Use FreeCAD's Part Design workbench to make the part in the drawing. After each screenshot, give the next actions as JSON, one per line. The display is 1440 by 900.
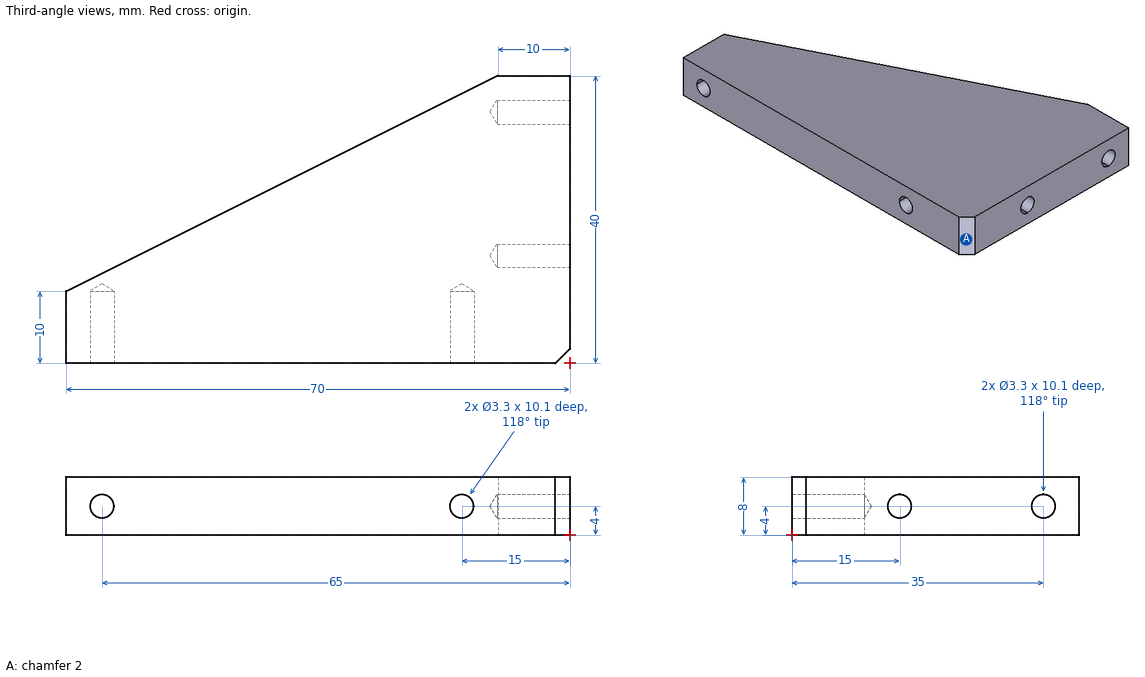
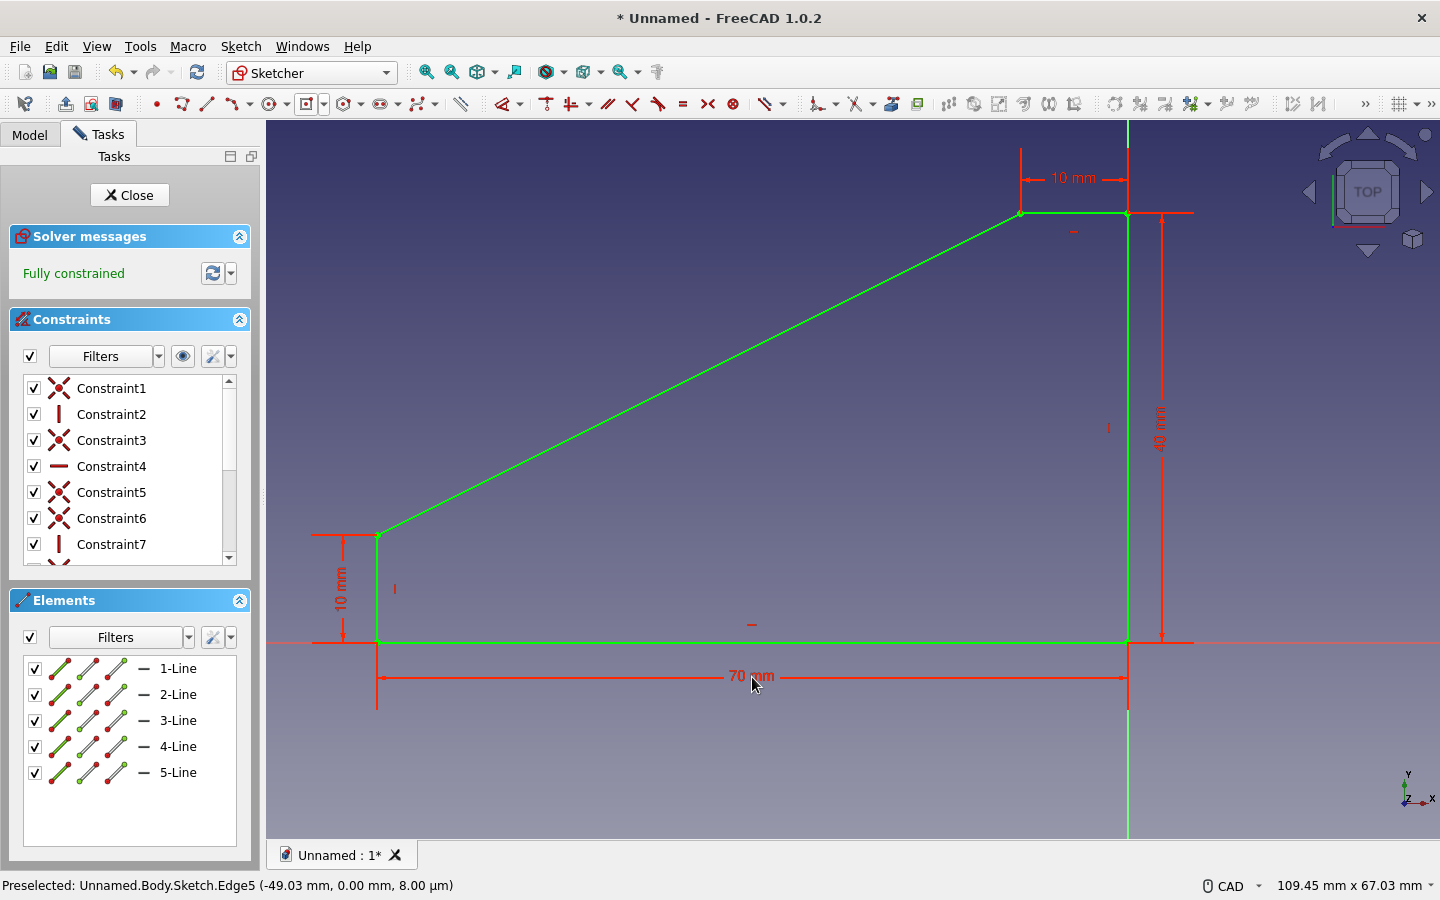
{"action": "left_click", "coordinate": [130, 195]}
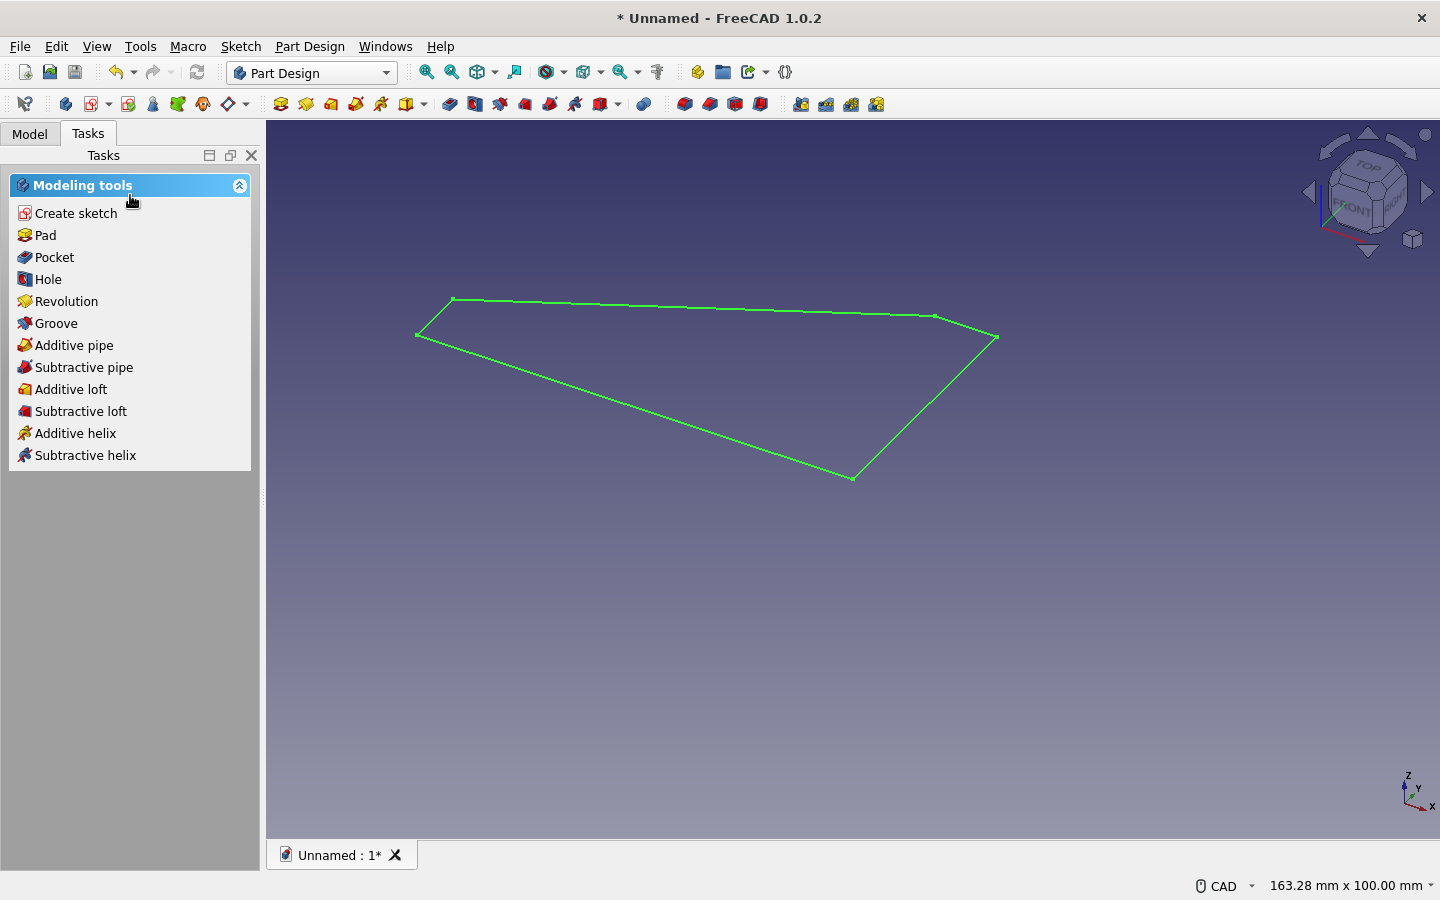
{"action": "left_click", "coordinate": [281, 104]}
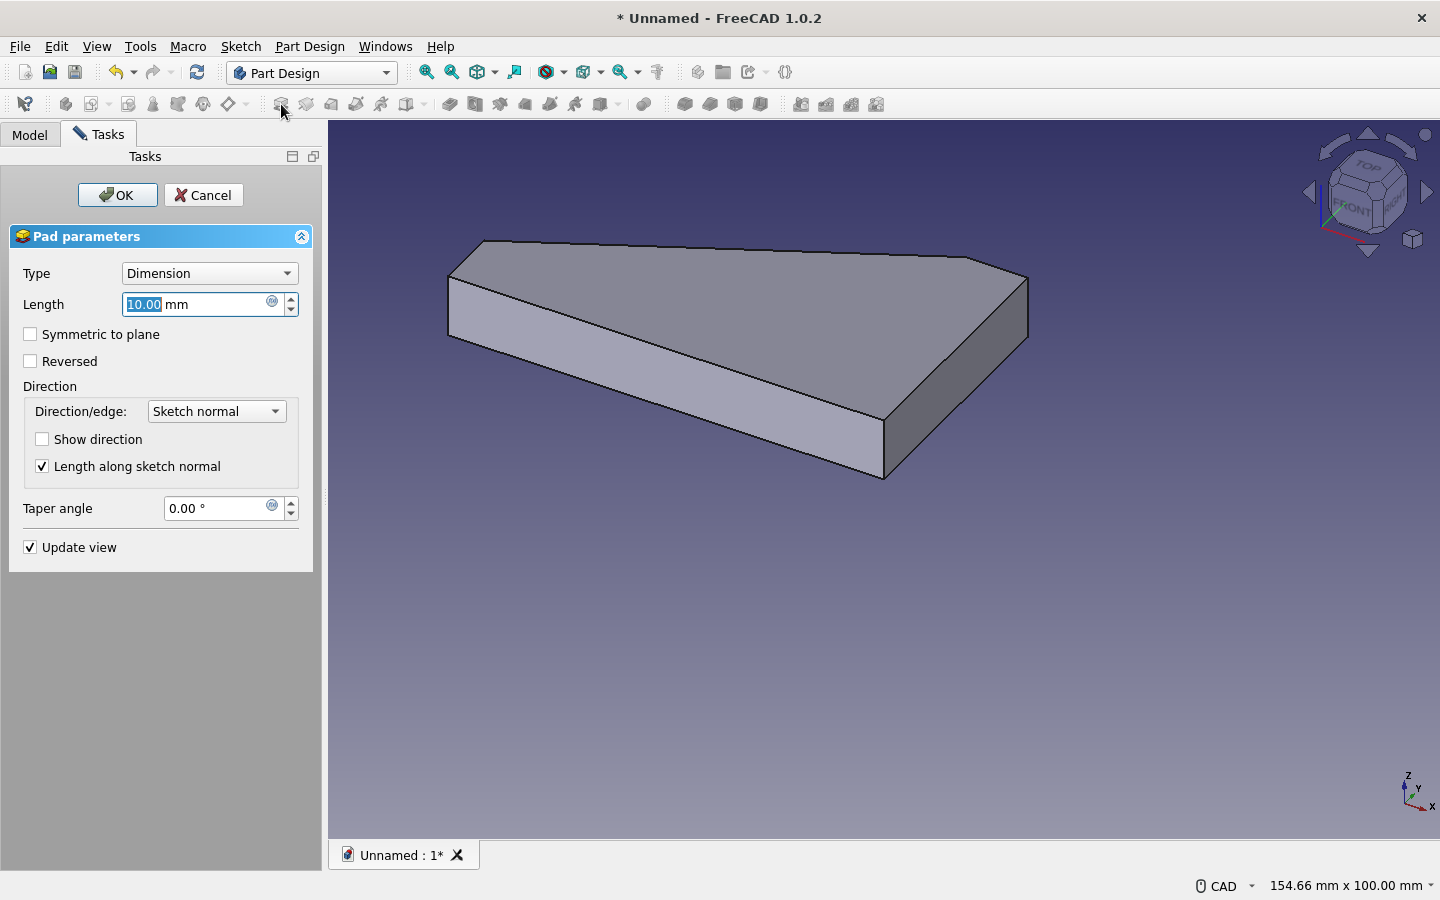
{"action": "type", "text": "8"}
{"action": "key", "text": "Tab"}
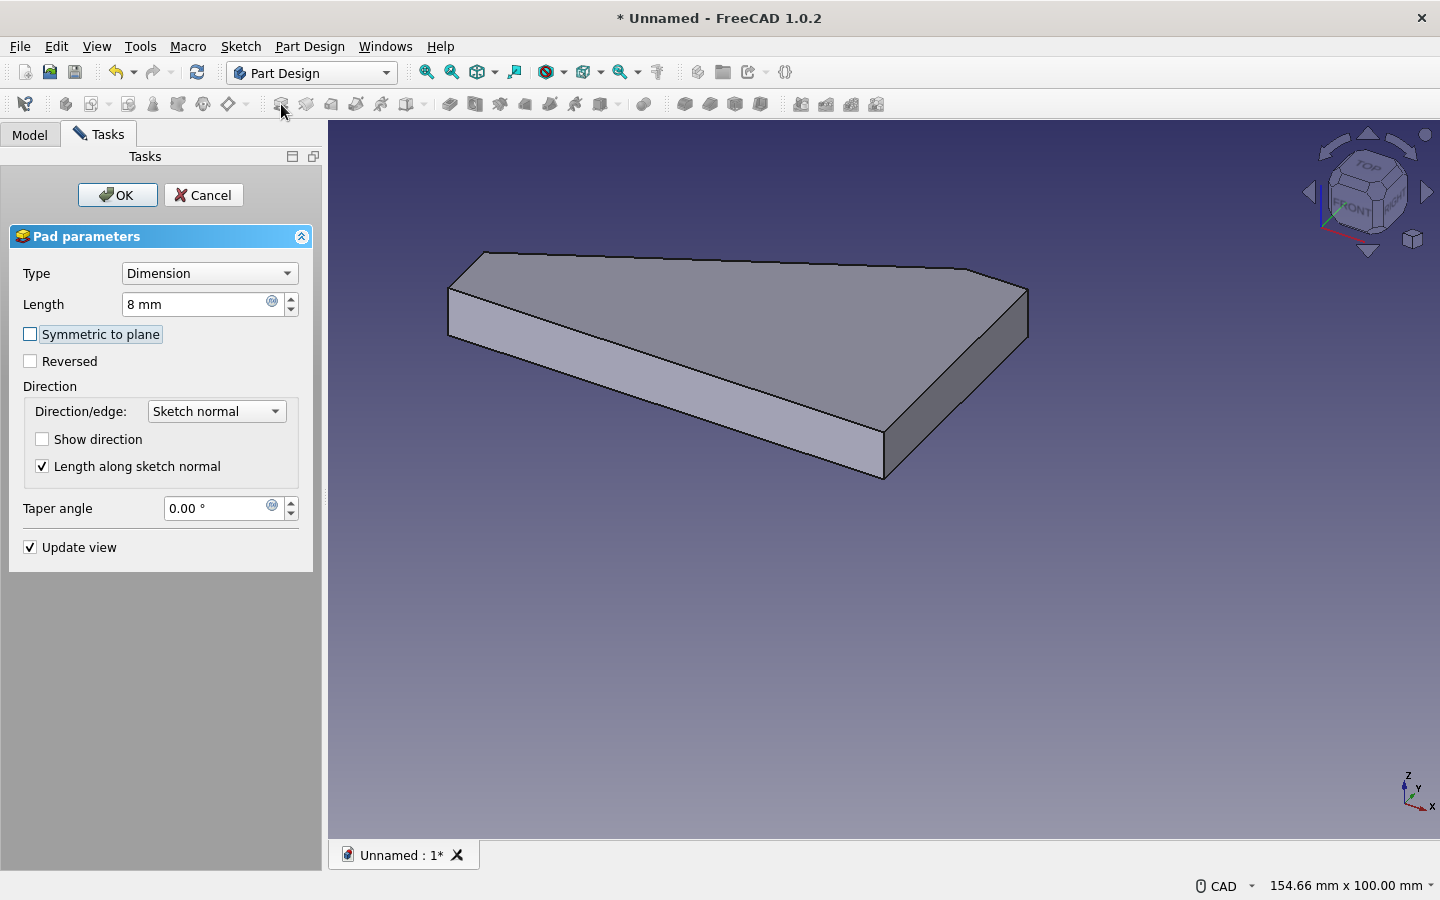
{"action": "left_click", "coordinate": [118, 195]}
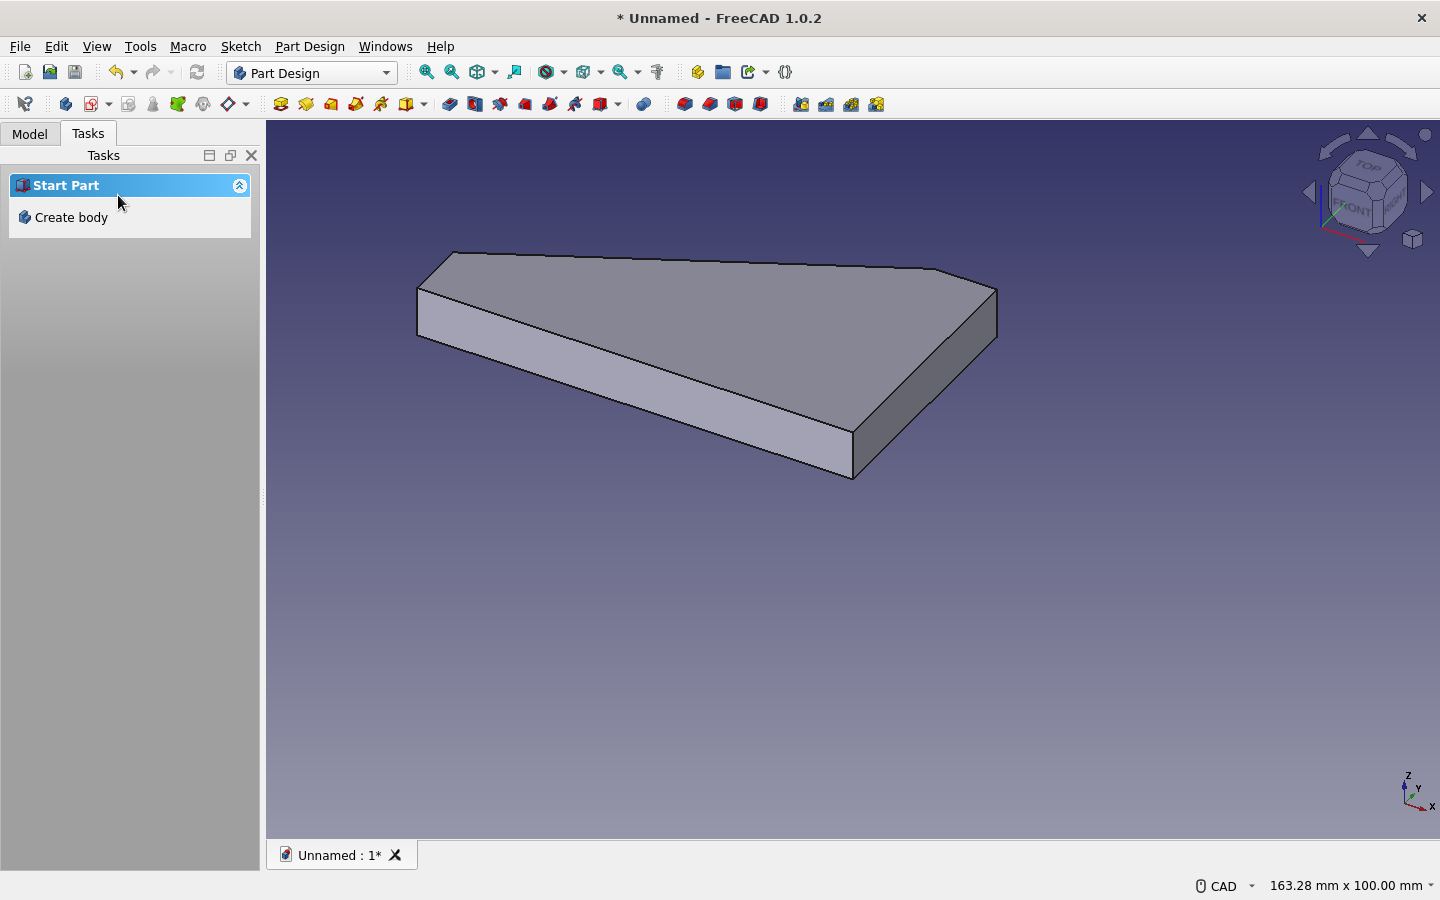
{"action": "left_click", "coordinate": [90, 104]}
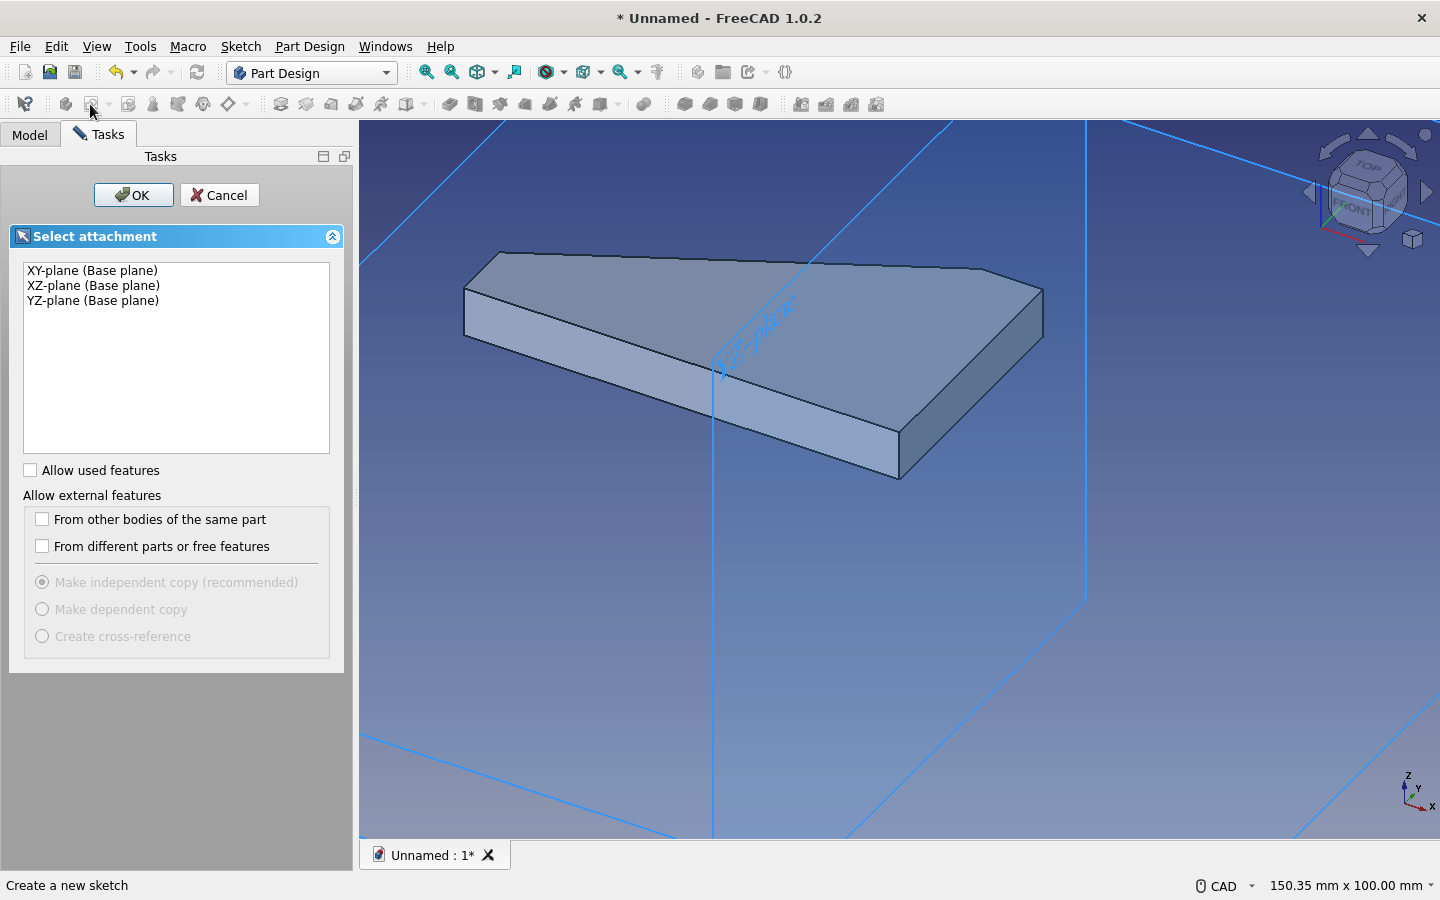
{"action": "left_click", "coordinate": [84, 286]}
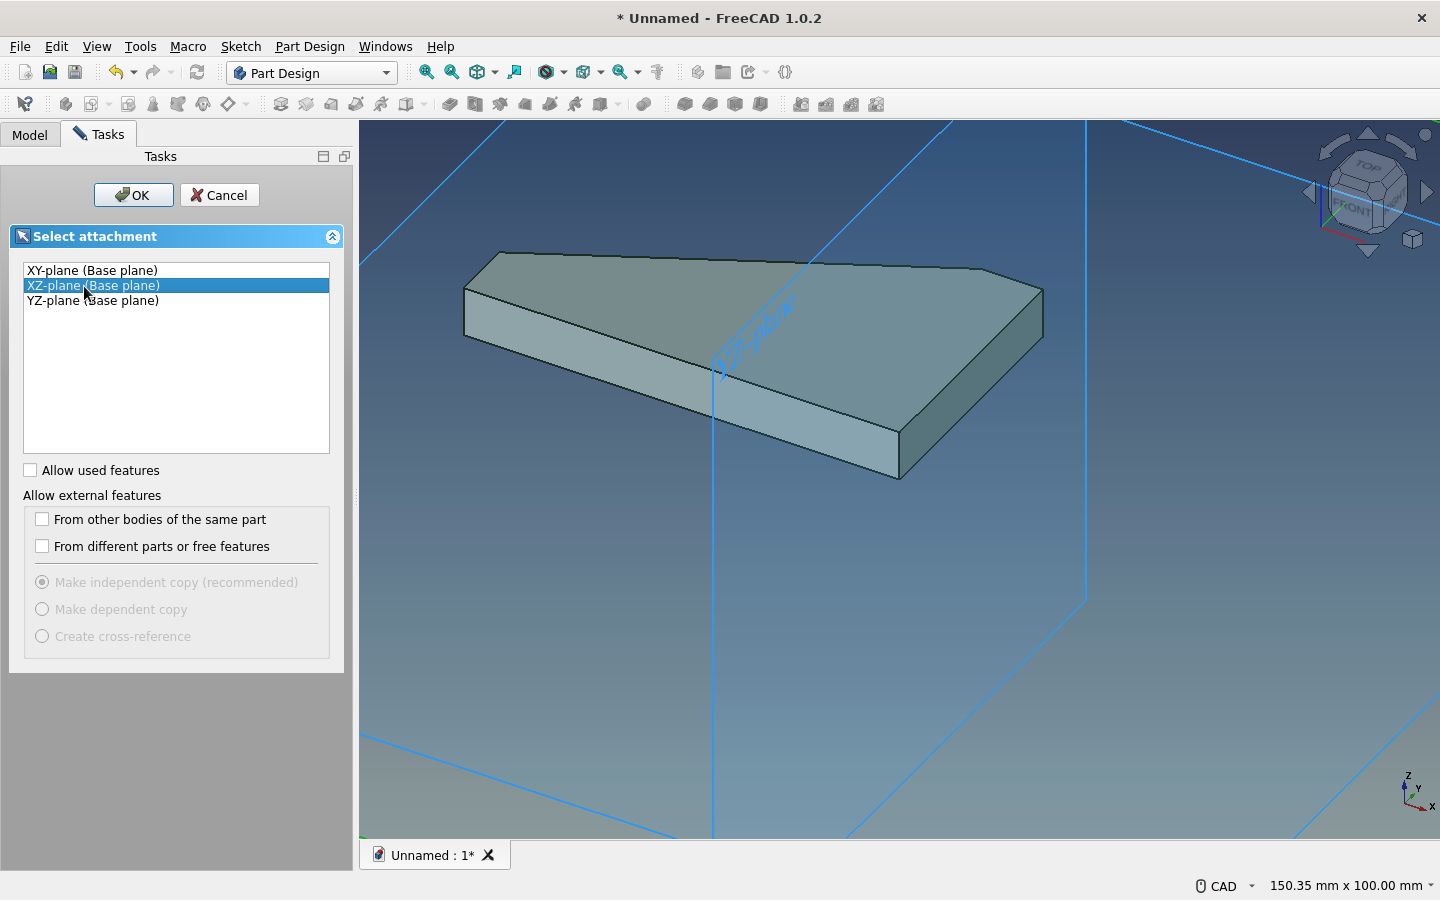
{"action": "left_click", "coordinate": [134, 195]}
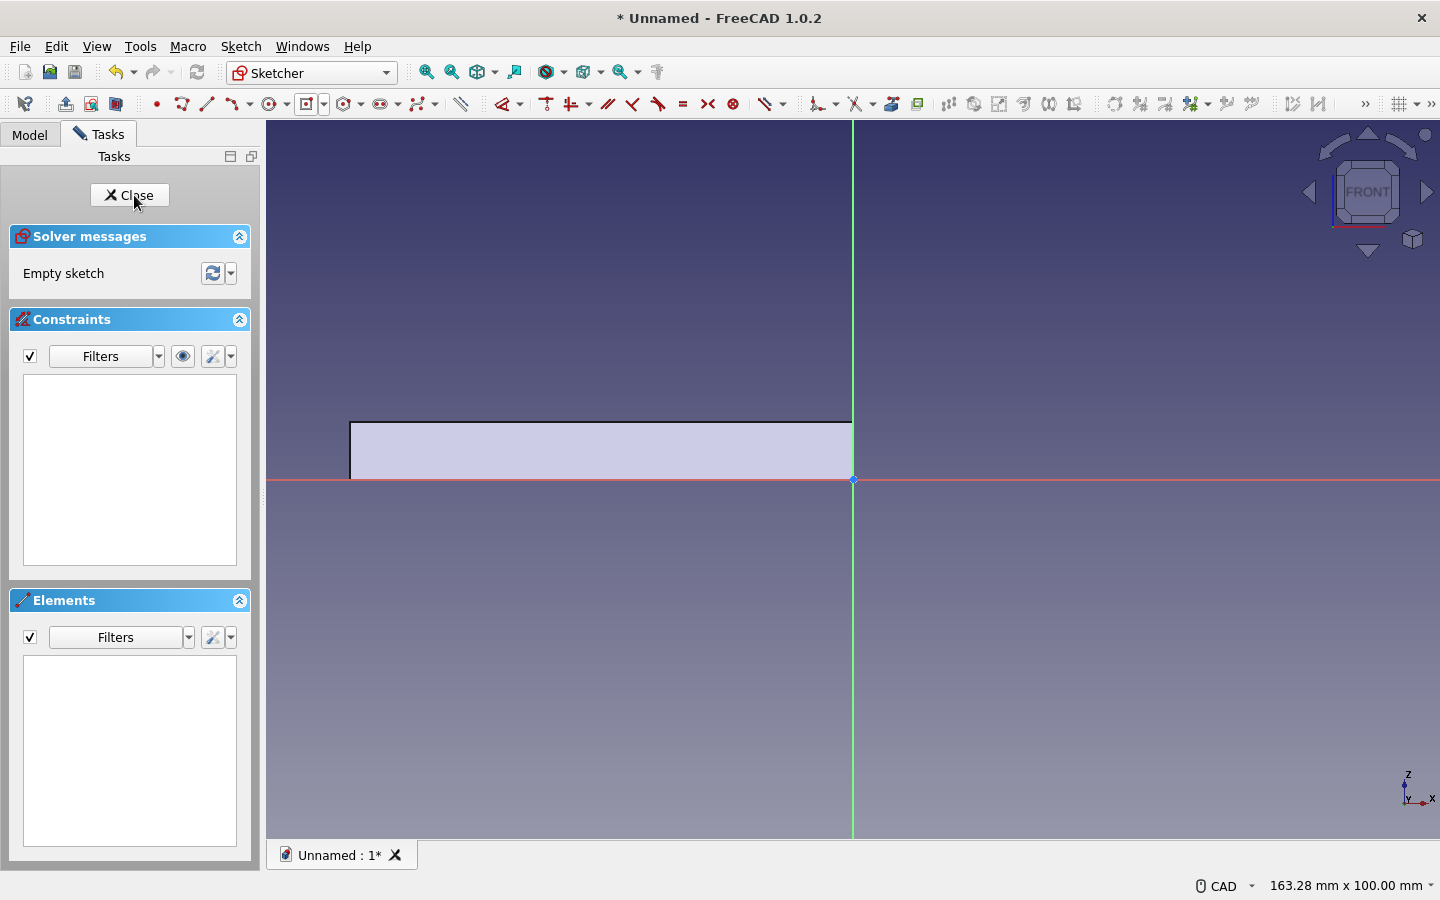
{"action": "scroll", "coordinate": [294, 418], "scroll_direction": "up", "scroll_amount": 2}